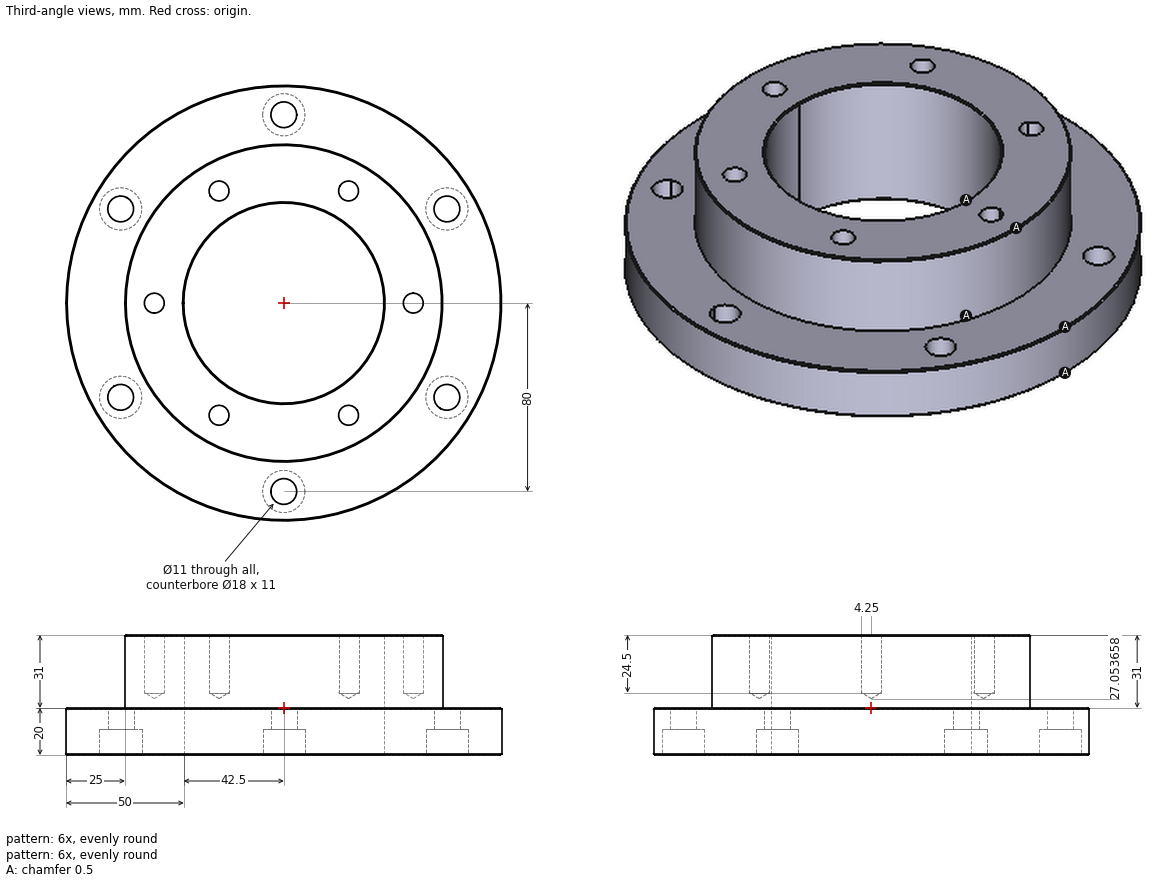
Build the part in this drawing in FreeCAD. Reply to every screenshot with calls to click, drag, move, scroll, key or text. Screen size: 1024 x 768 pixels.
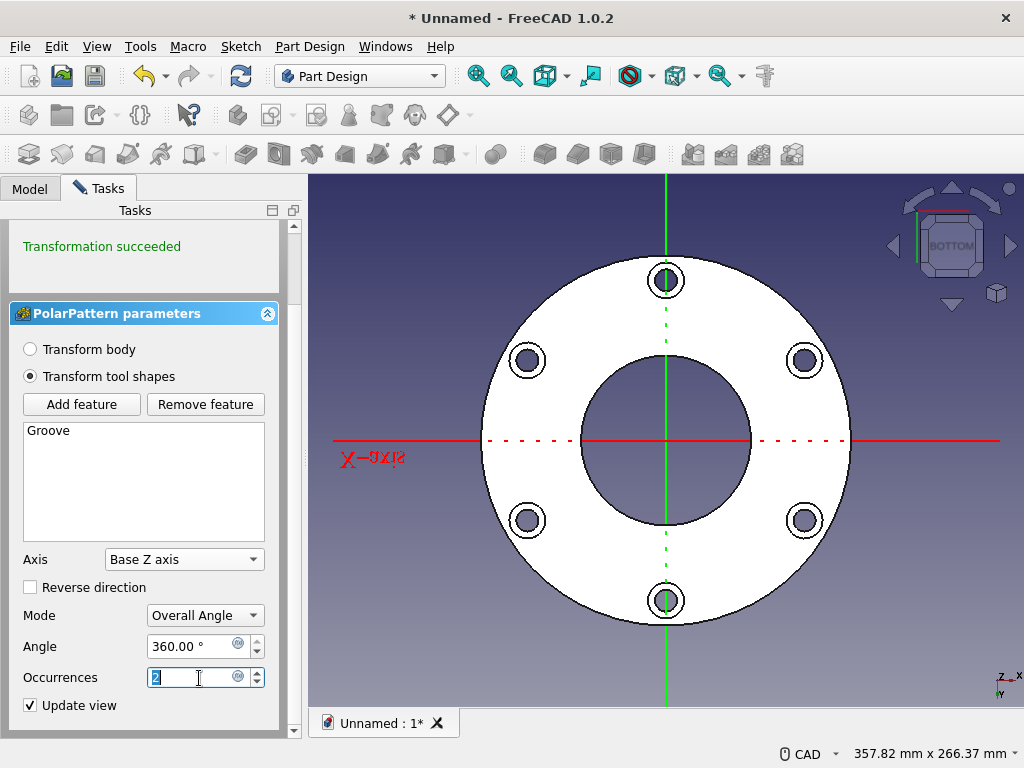
text(6)
key(Tab)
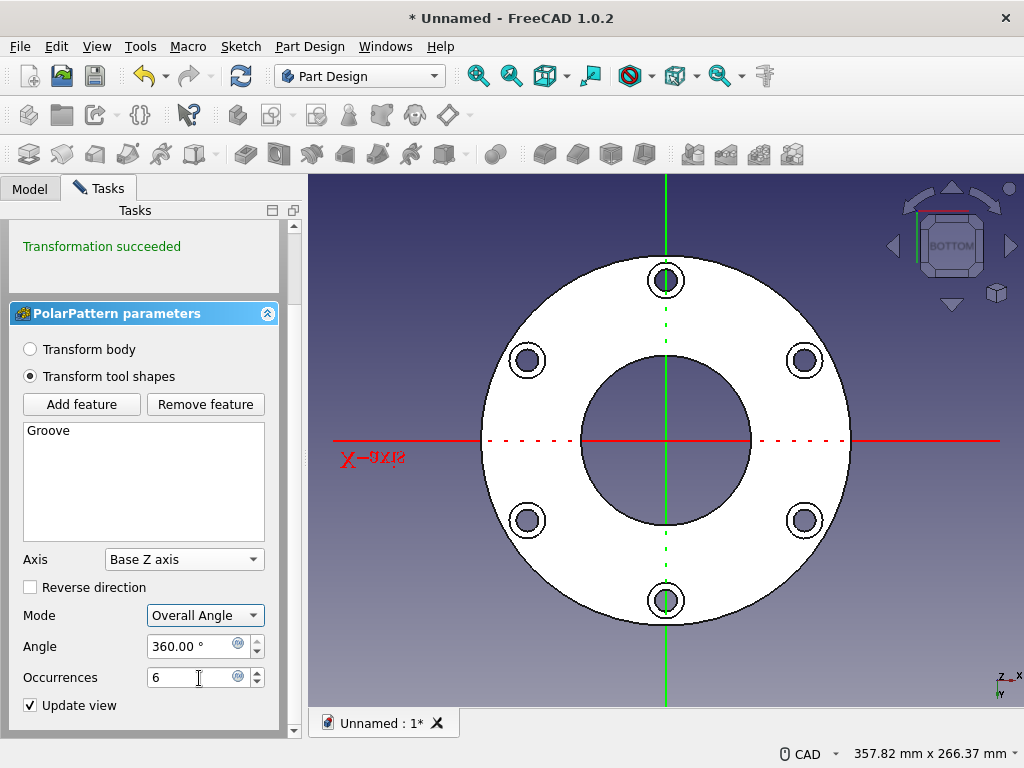
scroll(294, 479, up, 3)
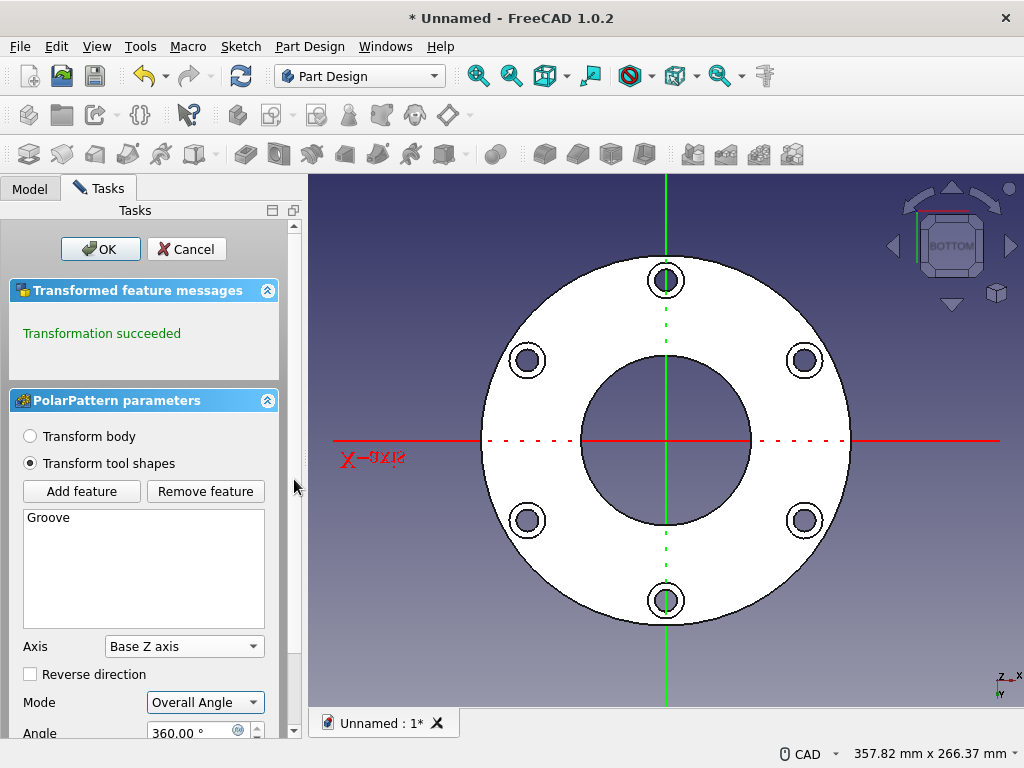
click(101, 249)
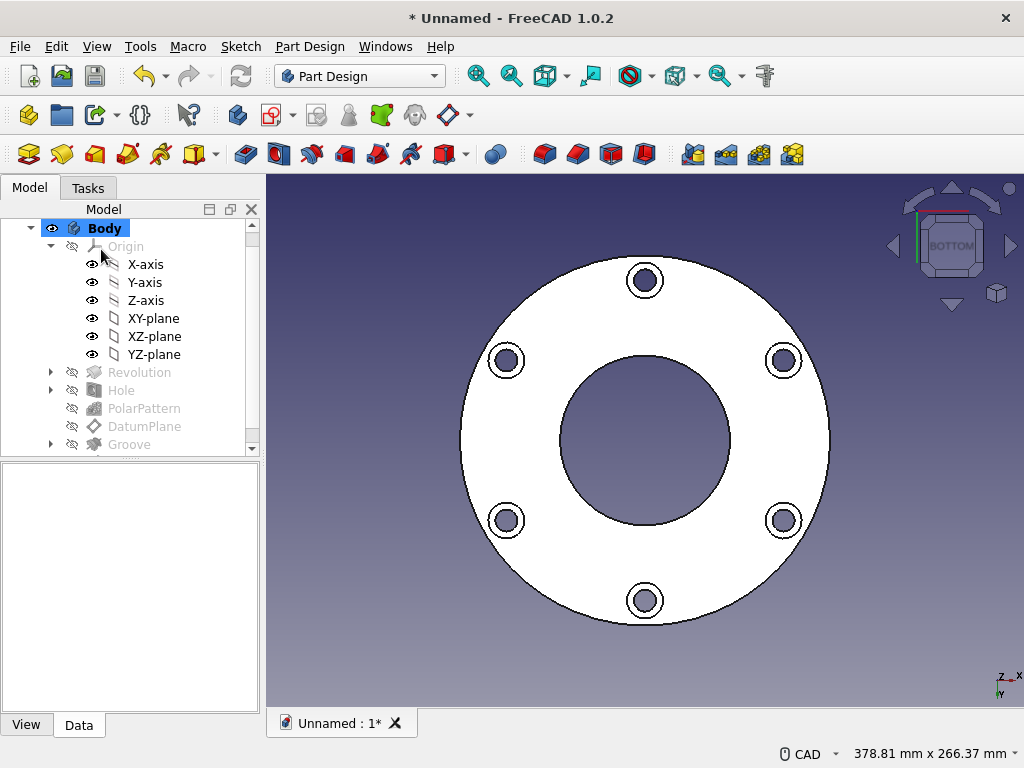
click(730, 440)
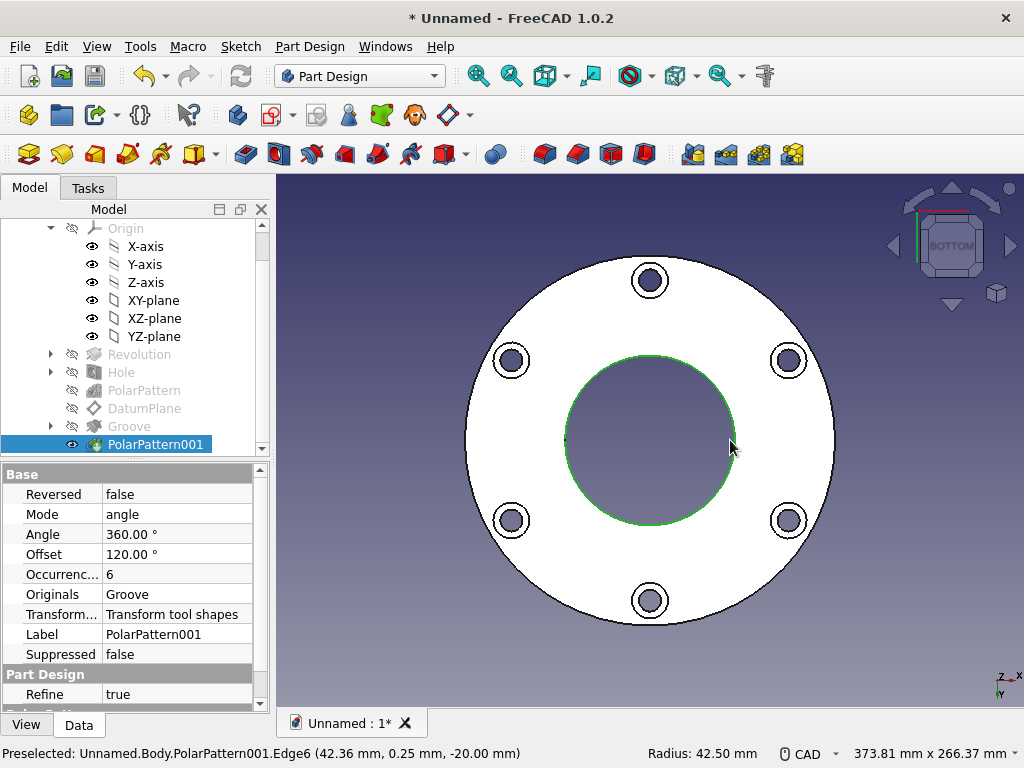
click(835, 440, ctrl)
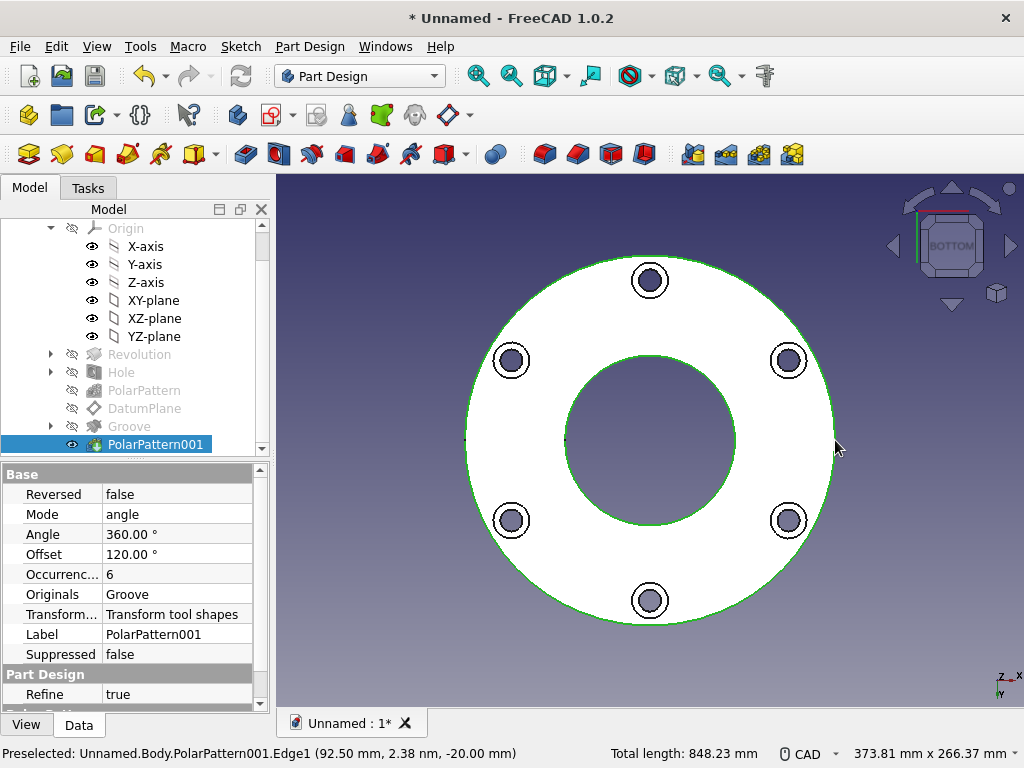
key(0)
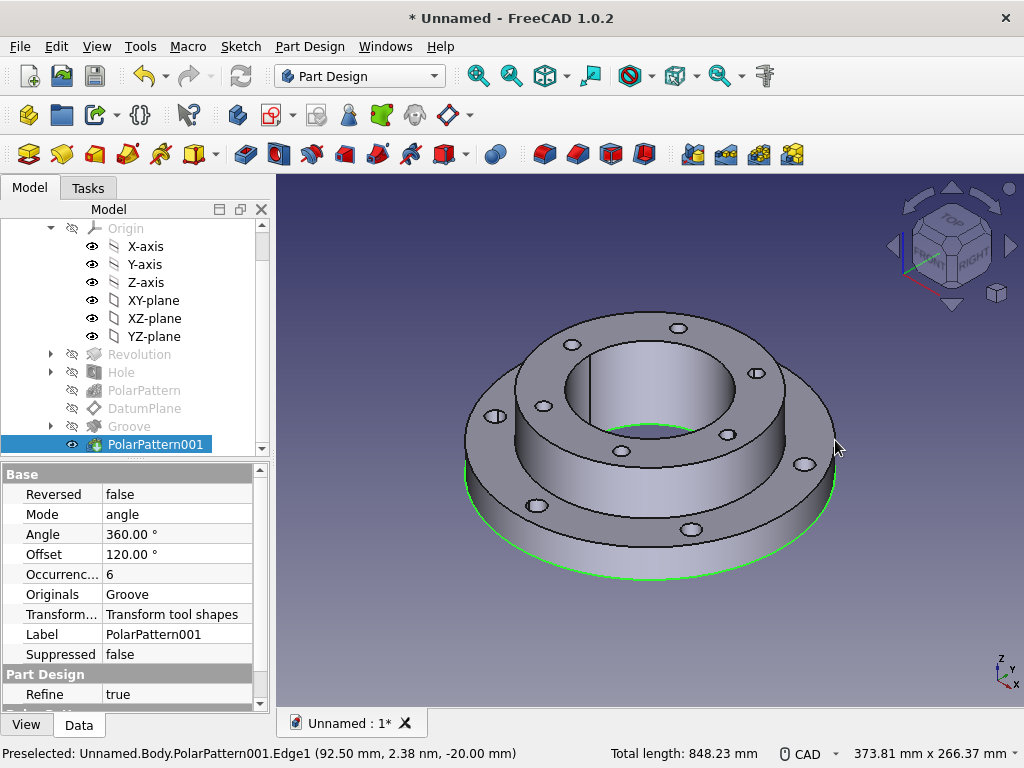
click(726, 367, ctrl)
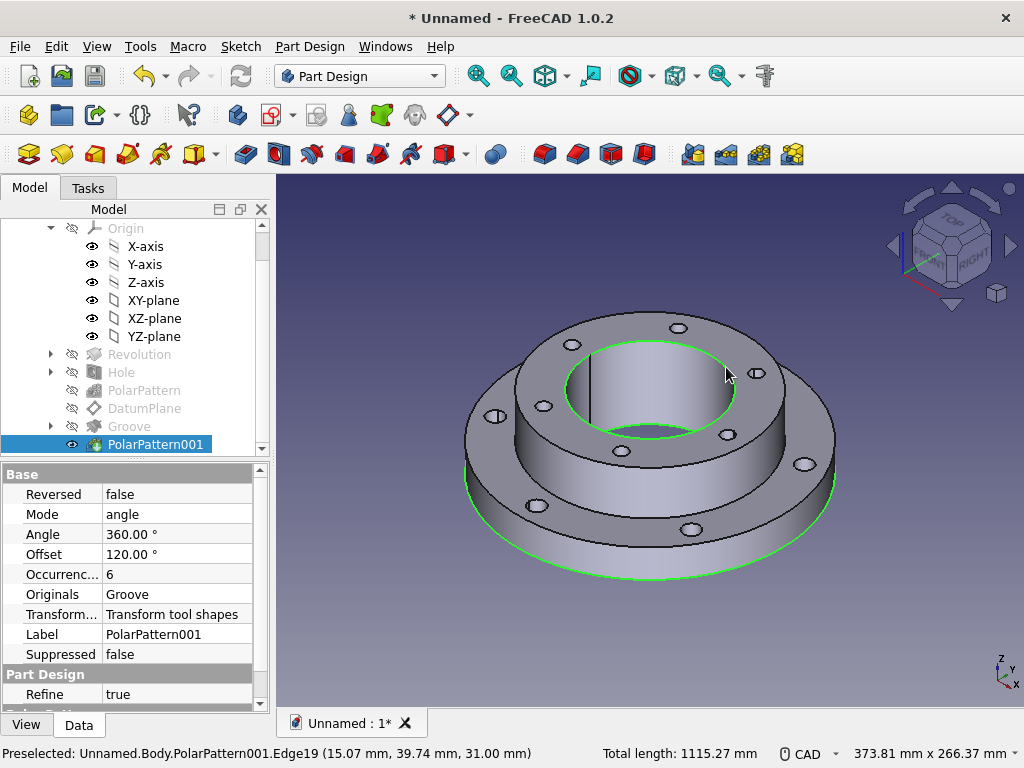
click(781, 515, ctrl)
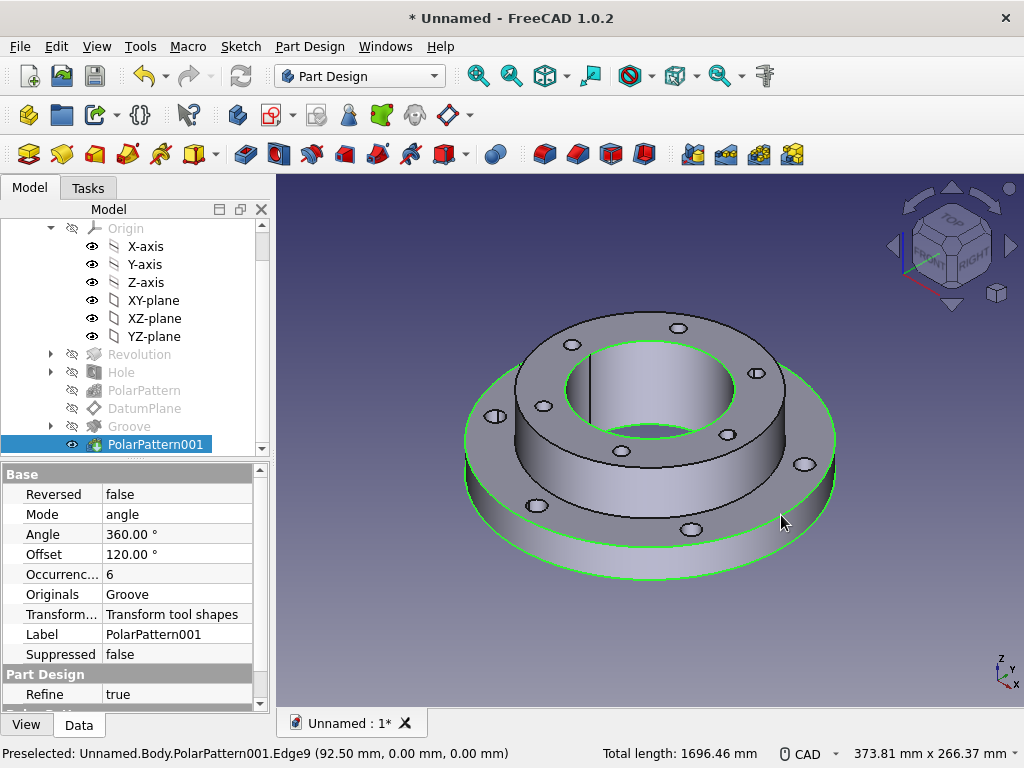
click(746, 444, ctrl)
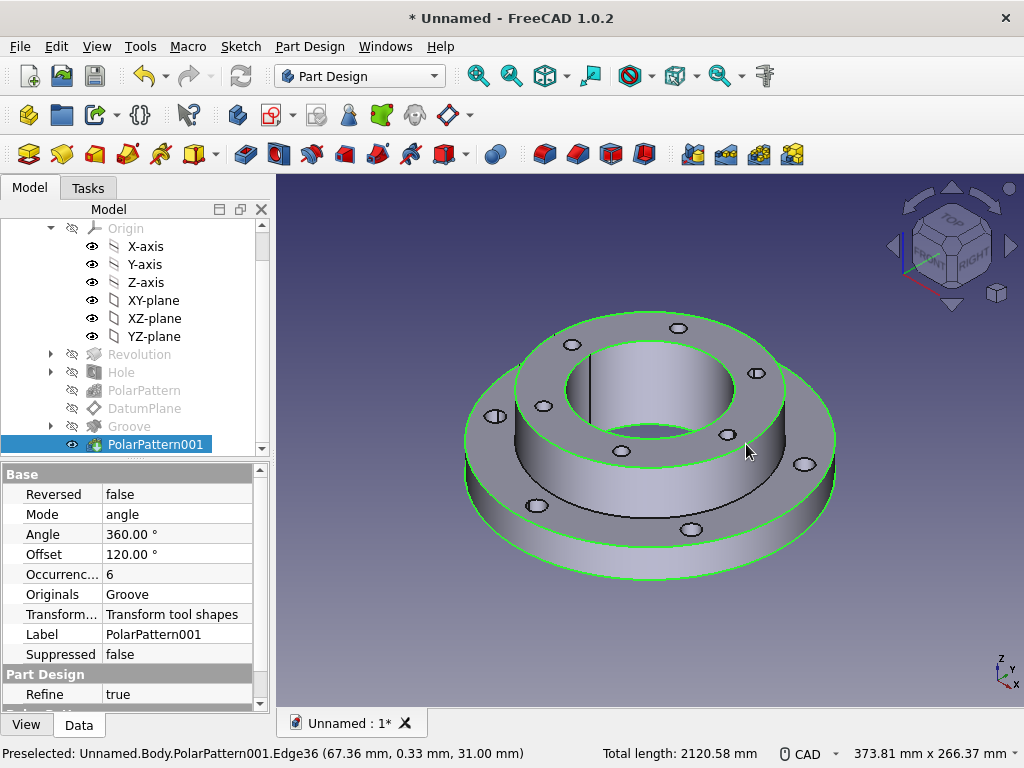
click(578, 154)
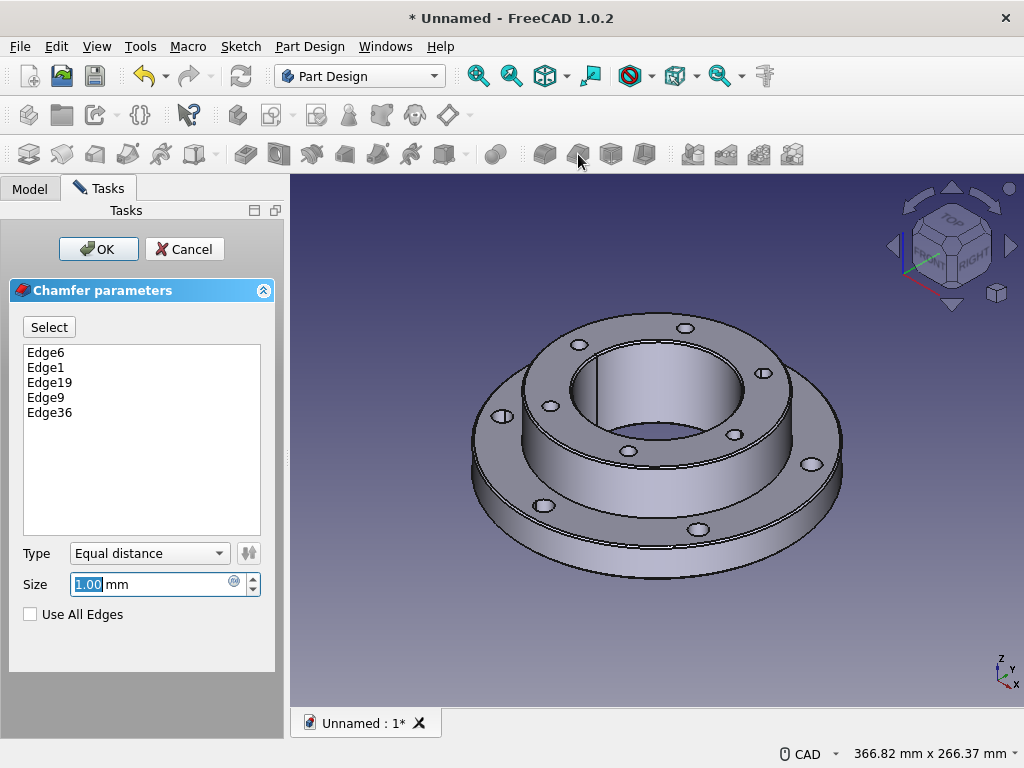
text(0.5)
key(Tab)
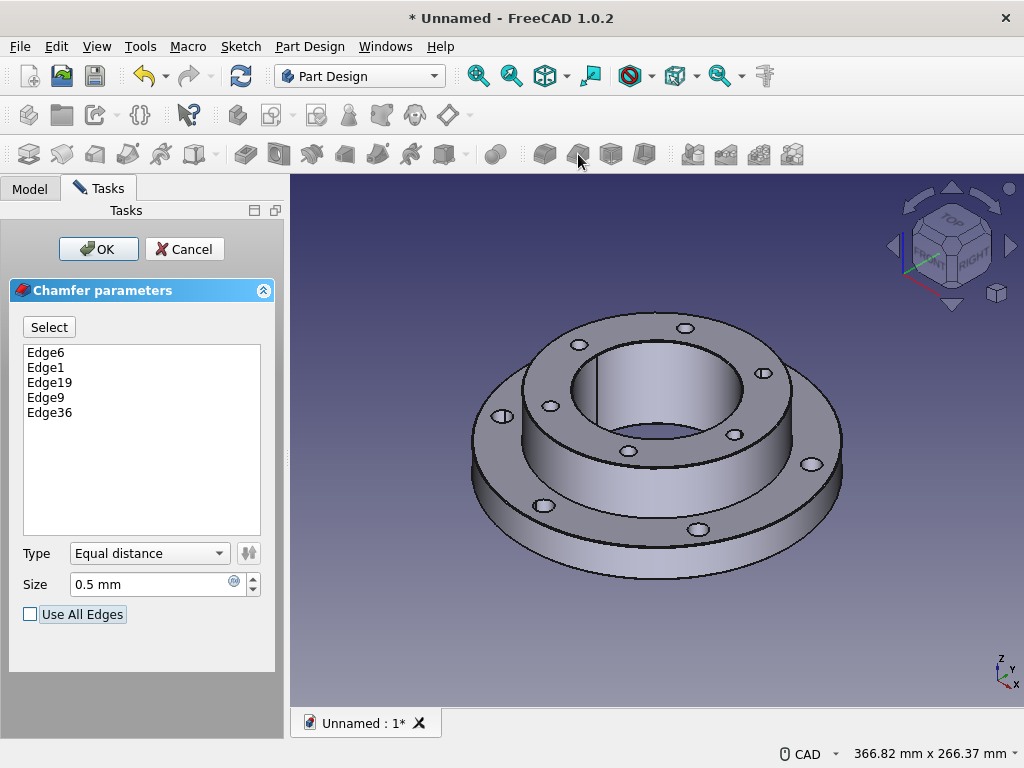
click(99, 249)